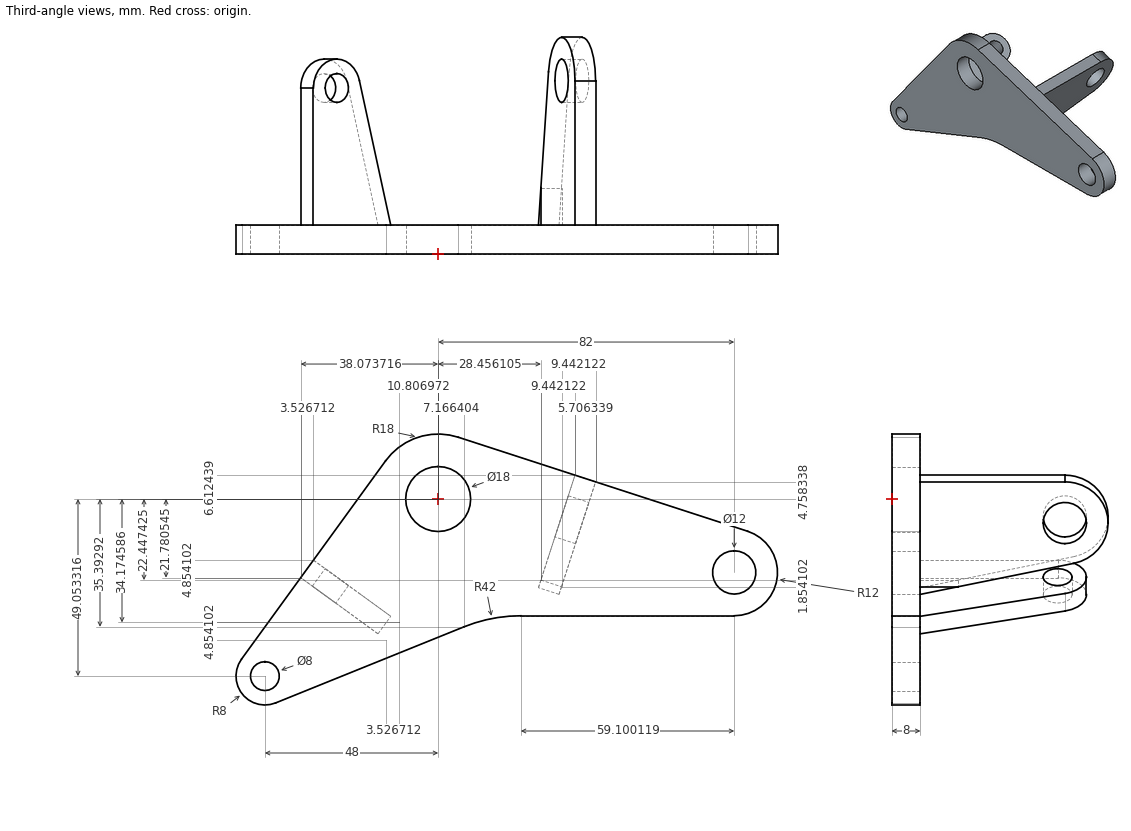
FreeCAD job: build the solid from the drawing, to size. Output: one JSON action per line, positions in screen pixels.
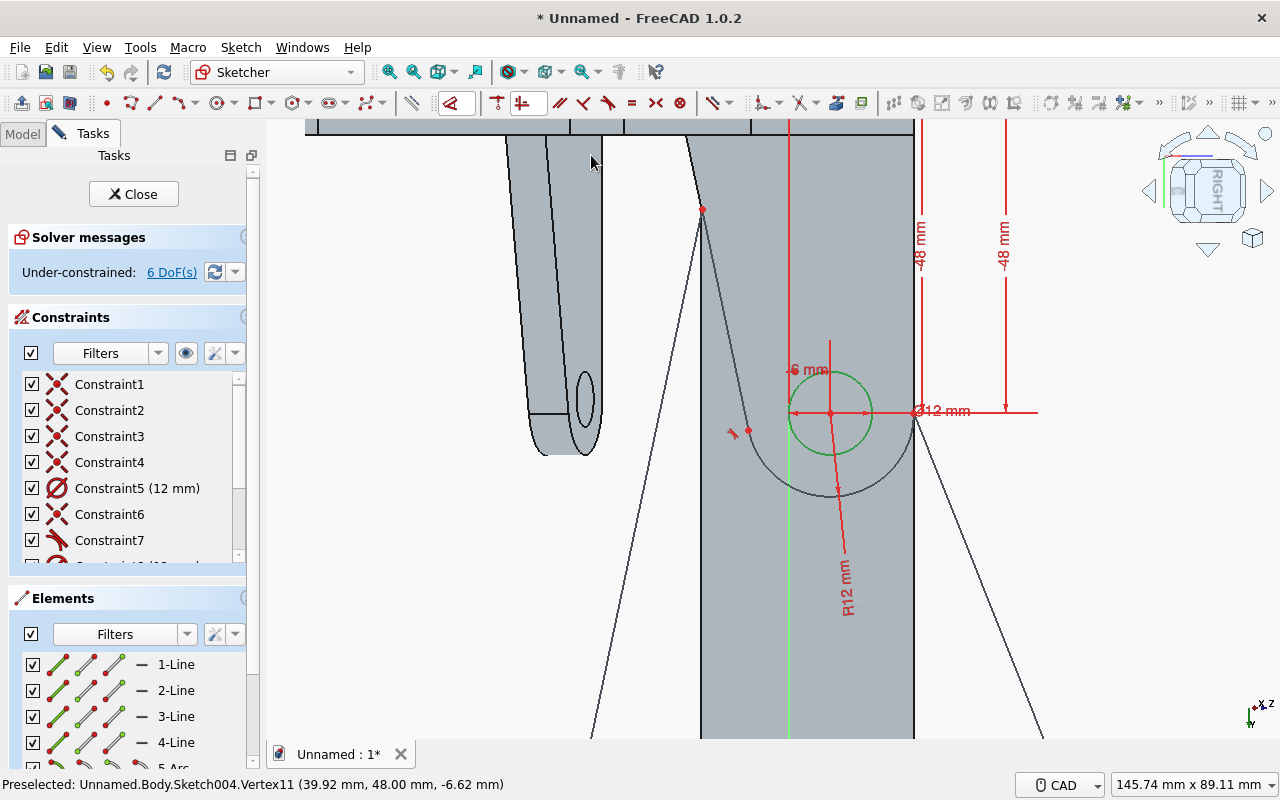
{"action": "scroll", "coordinate": [749, 430], "scroll_direction": "up", "scroll_amount": 5}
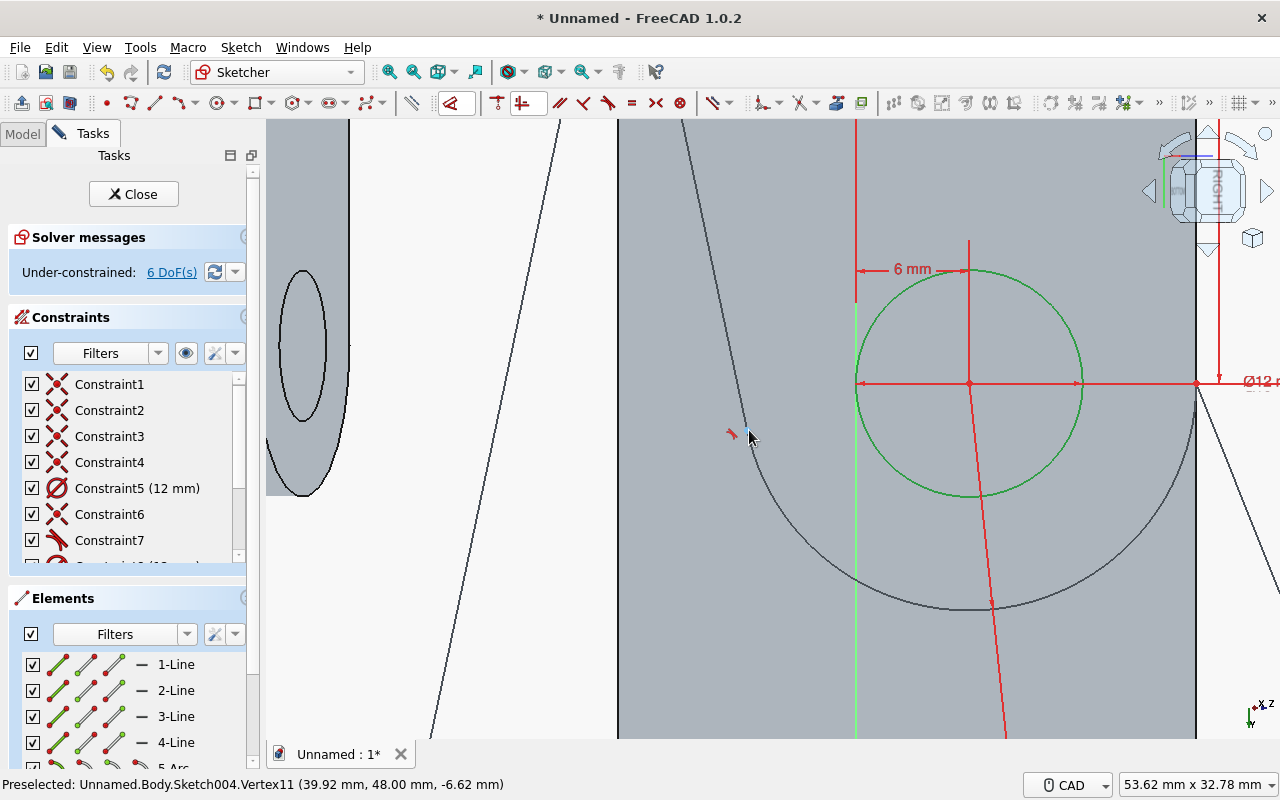
{"action": "left_click", "coordinate": [747, 430]}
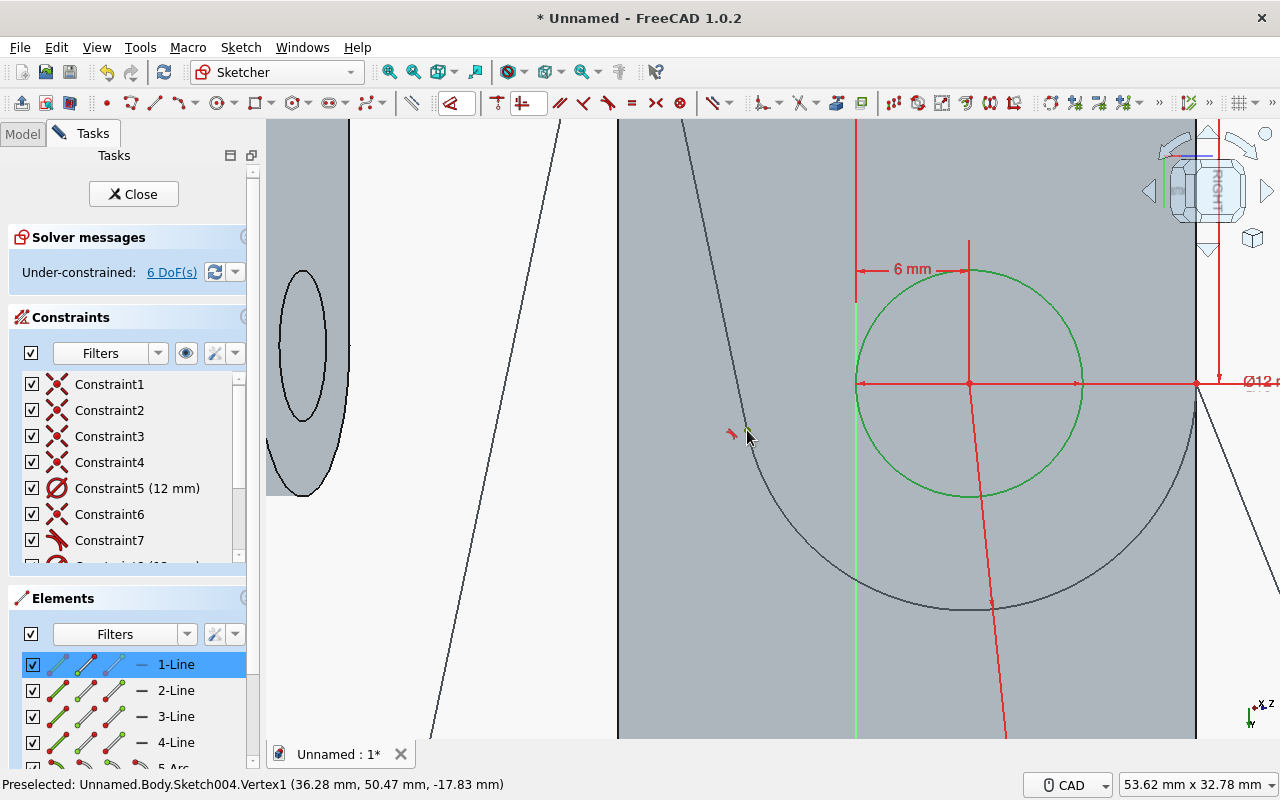
{"action": "left_click", "coordinate": [969, 384]}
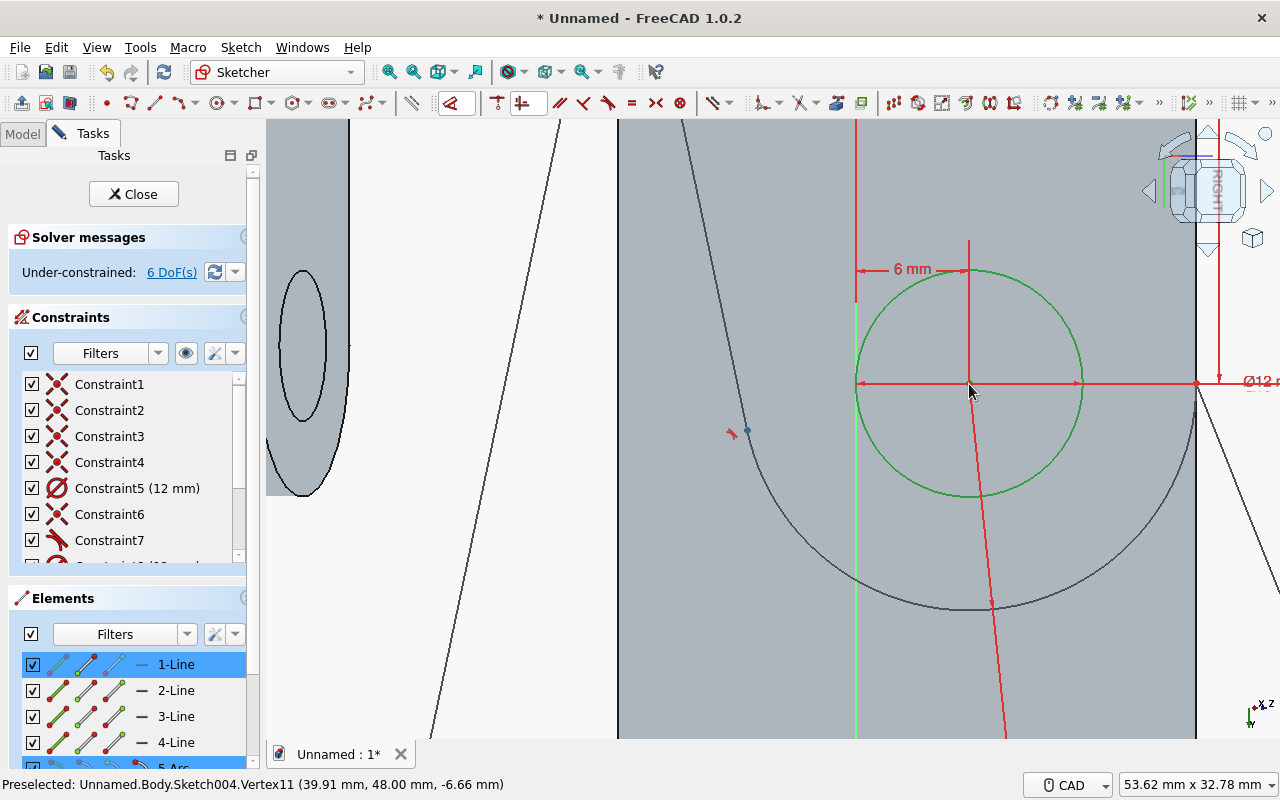
{"action": "key", "text": "i"}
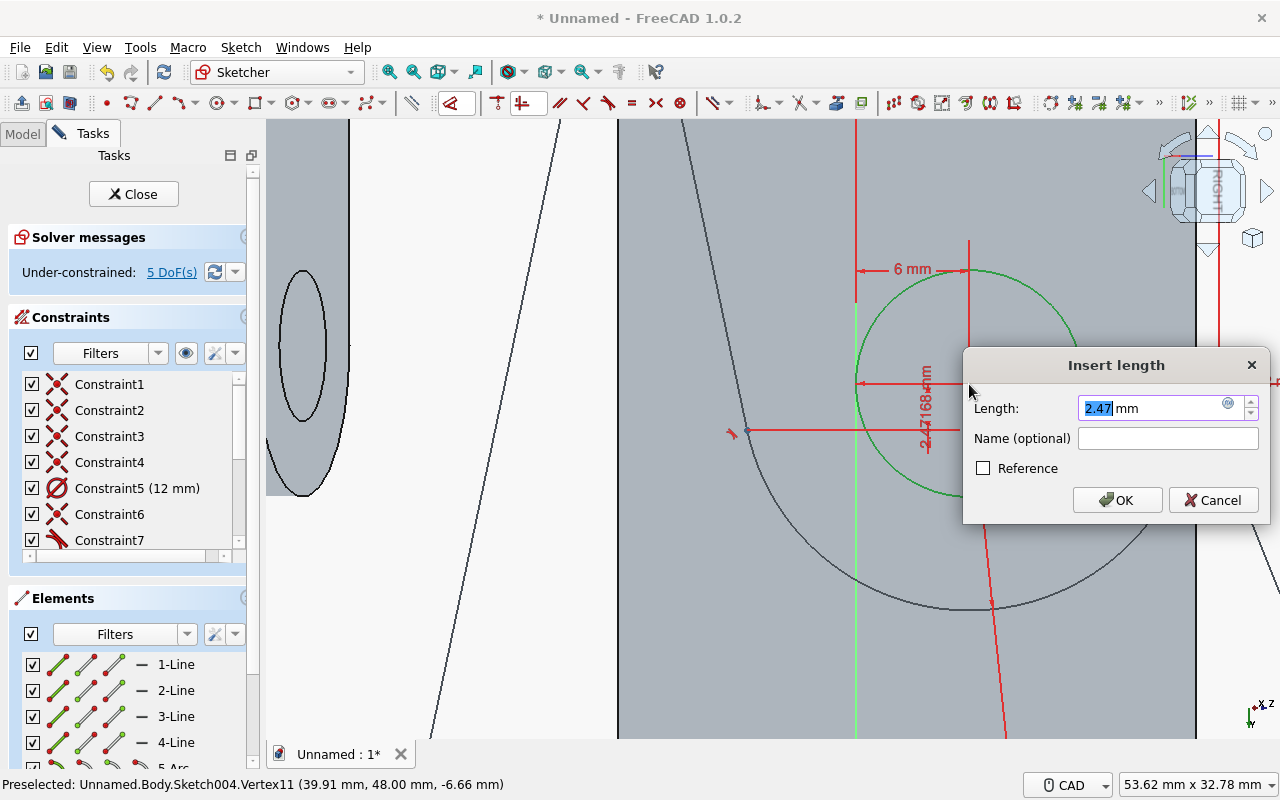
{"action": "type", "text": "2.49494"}
{"action": "key", "text": "Return"}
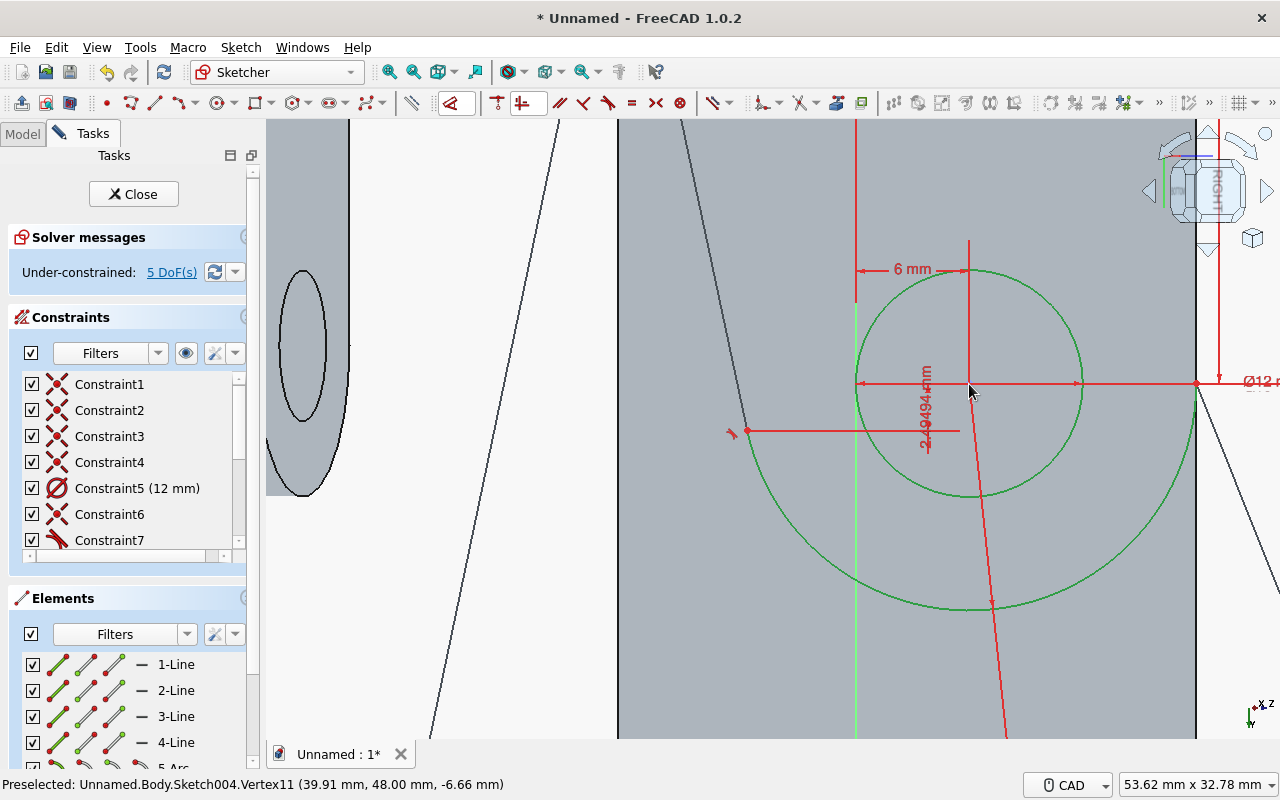
{"action": "scroll", "coordinate": [648, 393], "scroll_direction": "down", "scroll_amount": 9}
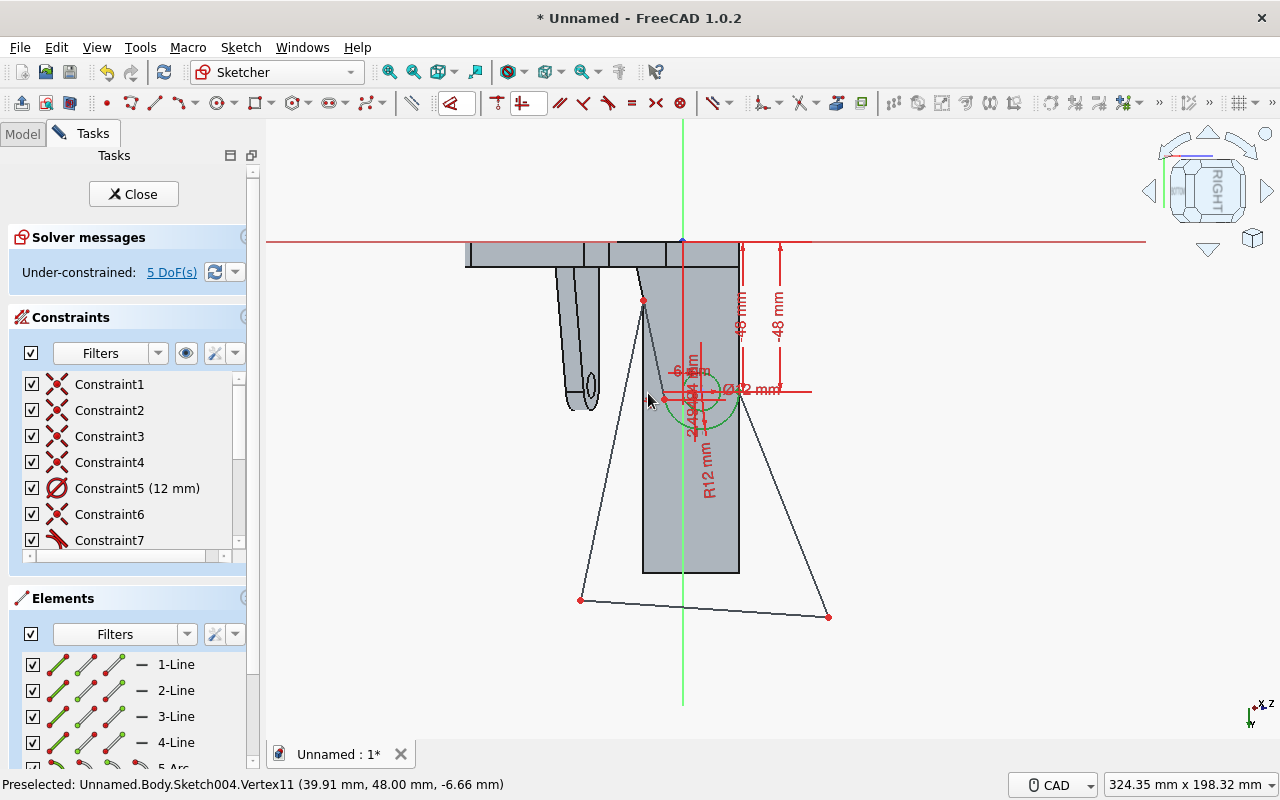
{"action": "left_click", "coordinate": [644, 300]}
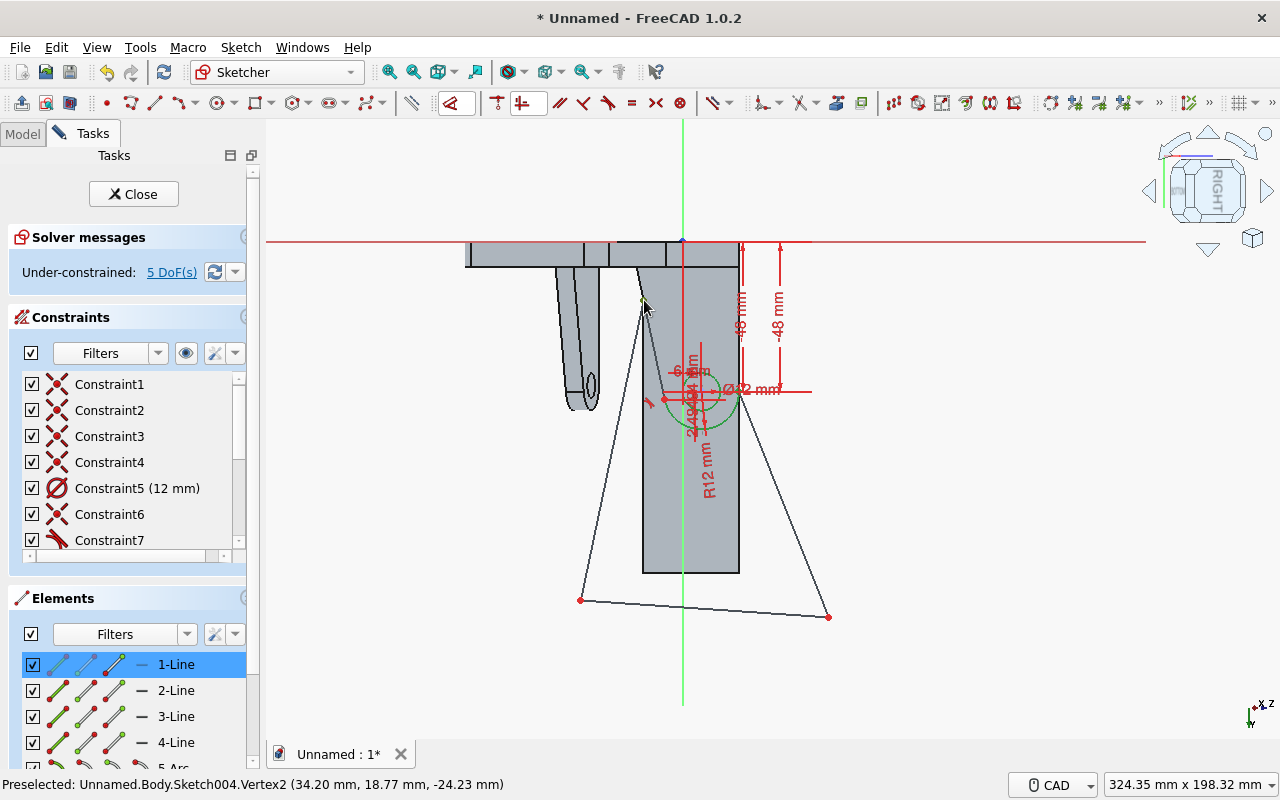
{"action": "key", "text": "l"}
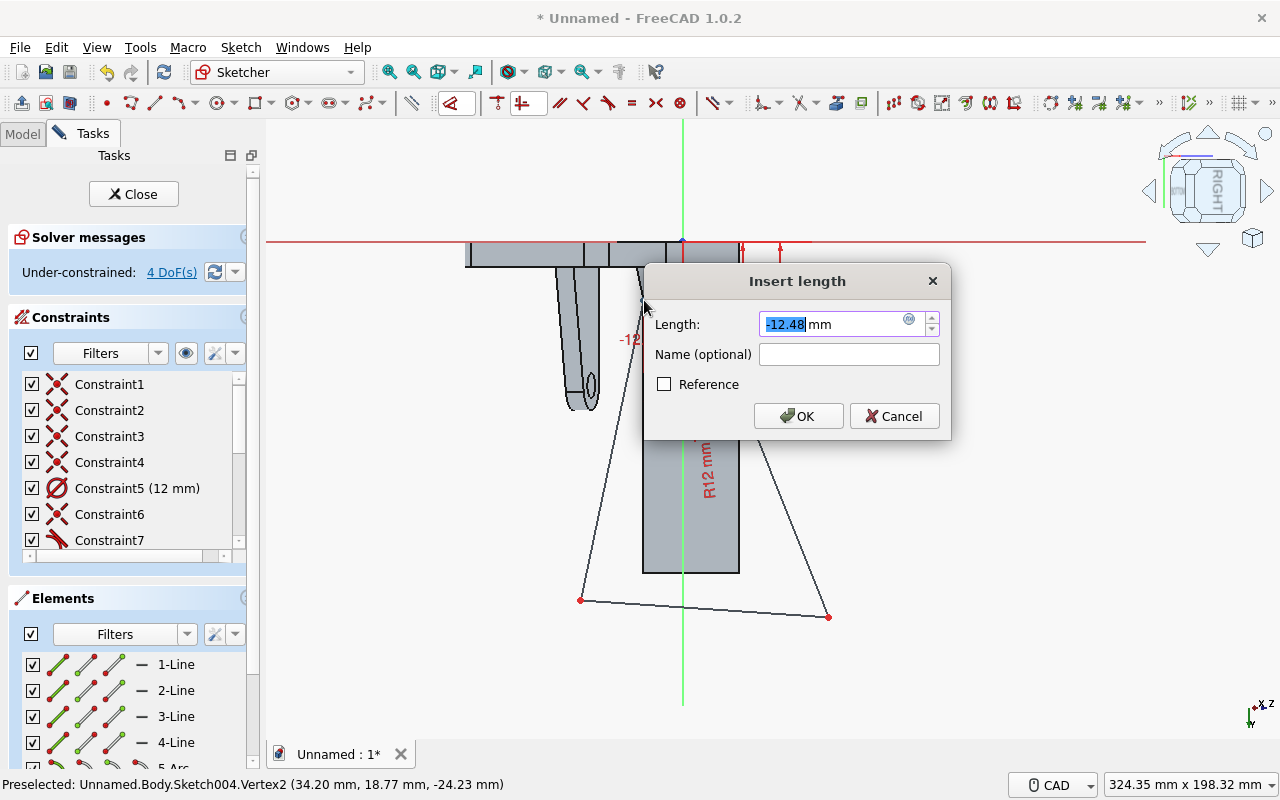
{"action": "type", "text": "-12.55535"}
{"action": "key", "text": "Return"}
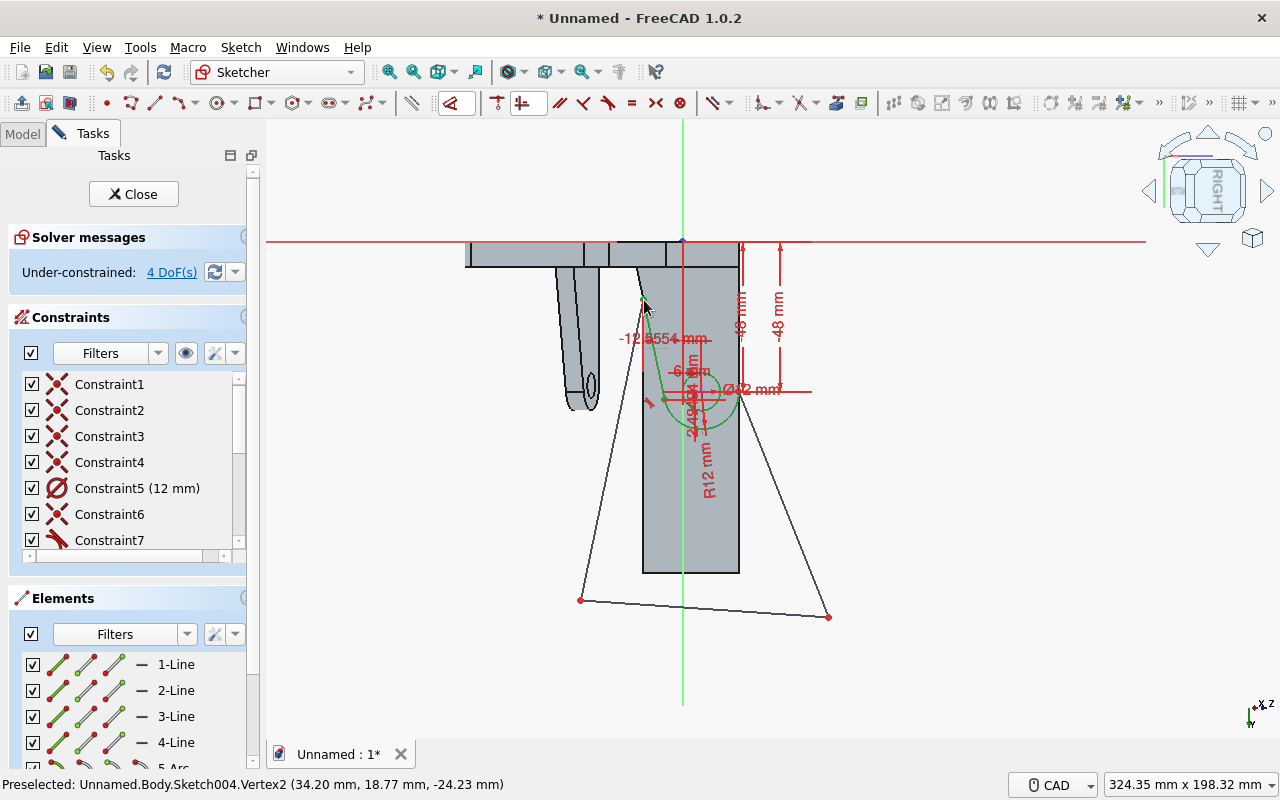
{"action": "scroll", "coordinate": [655, 606], "scroll_direction": "up", "scroll_amount": 5}